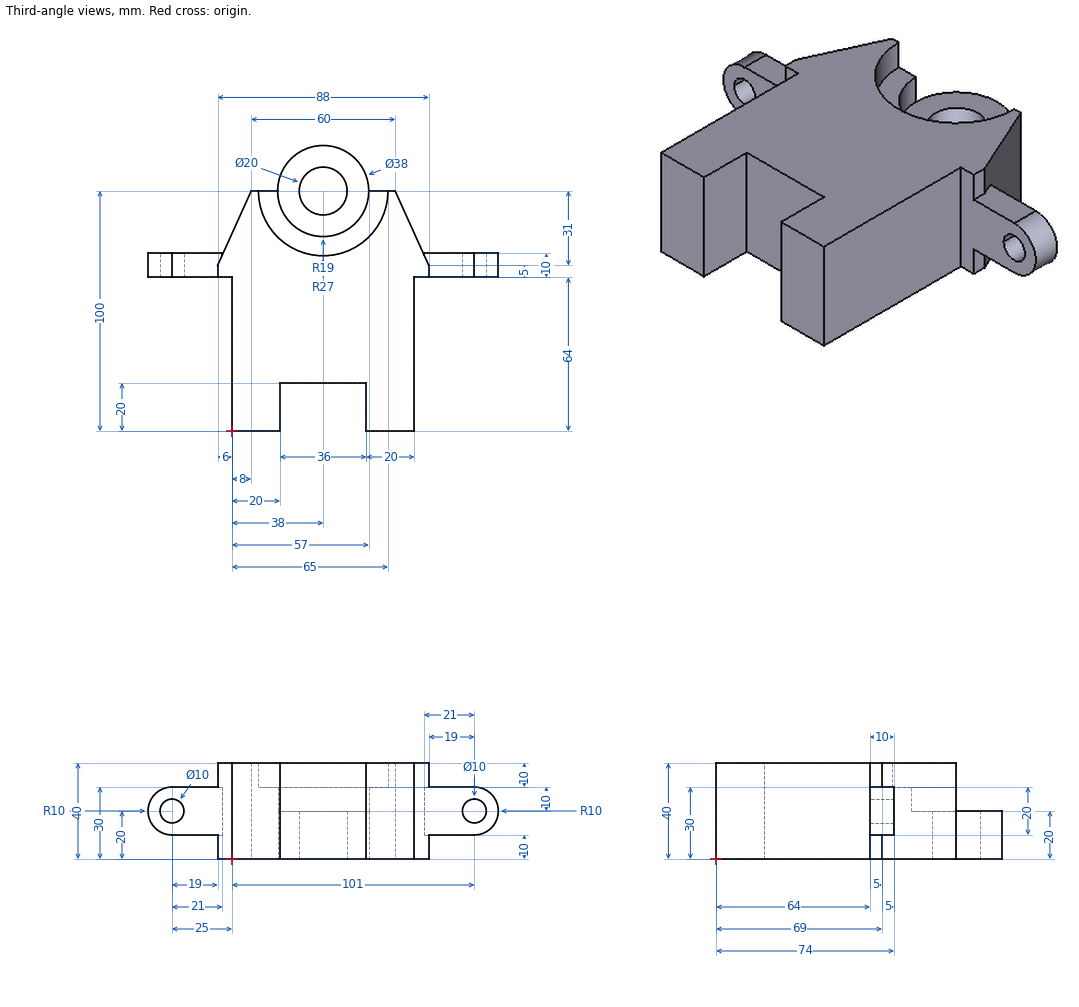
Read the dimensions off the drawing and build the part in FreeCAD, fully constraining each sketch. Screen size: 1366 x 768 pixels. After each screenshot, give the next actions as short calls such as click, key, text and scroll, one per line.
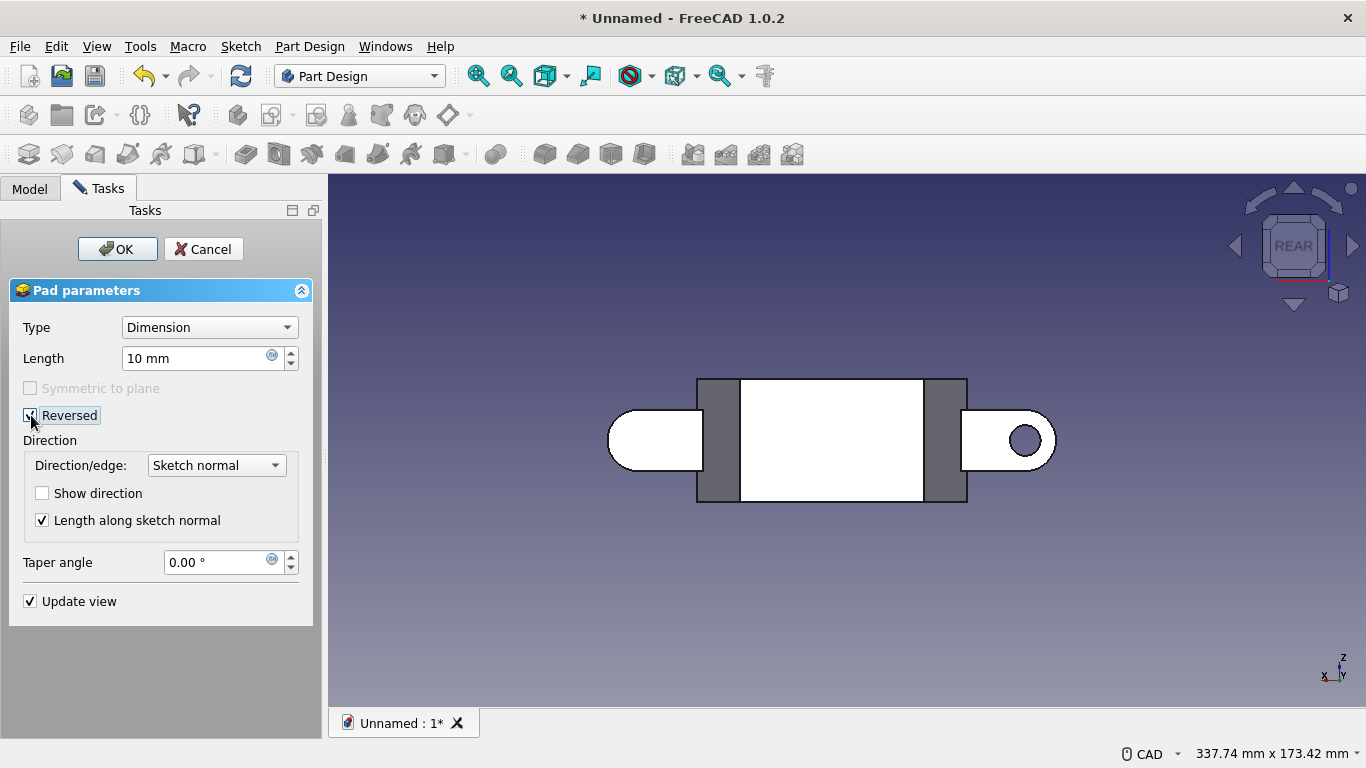
click(118, 249)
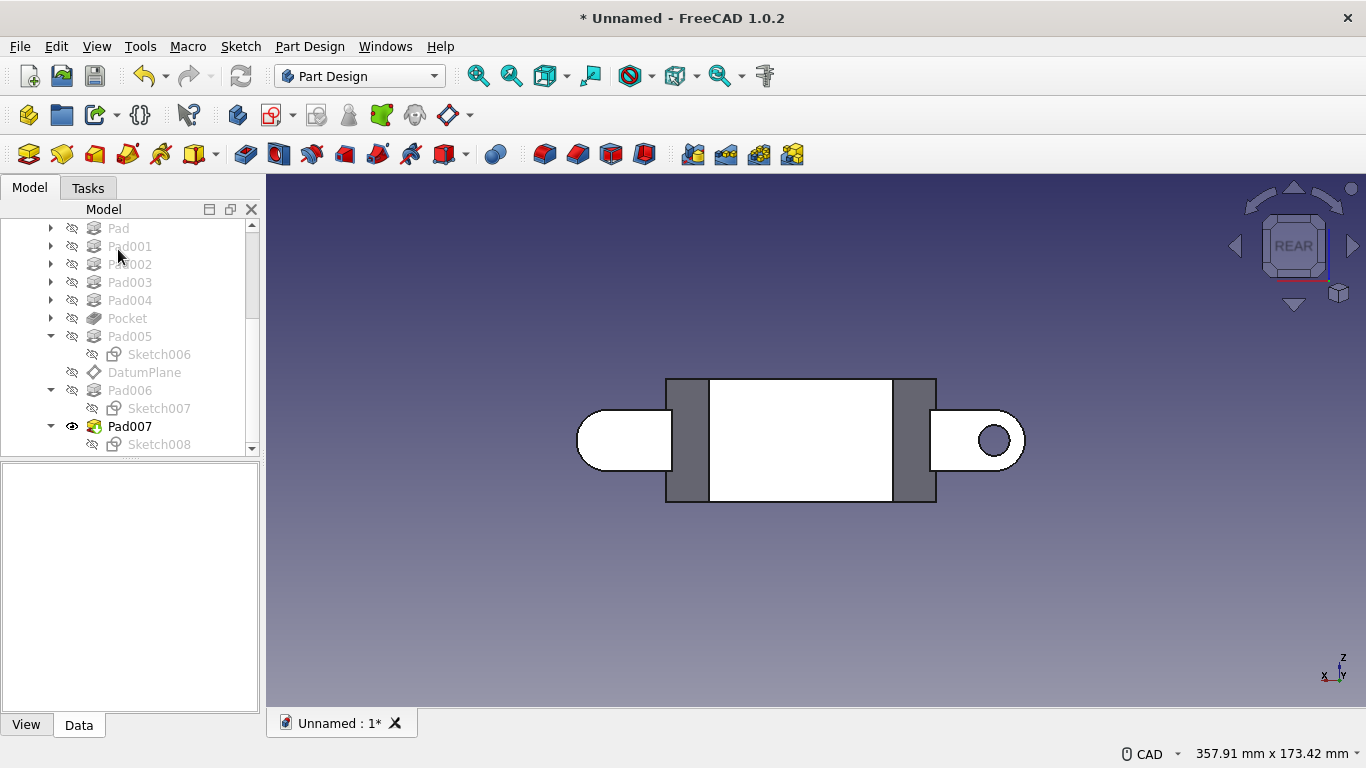
click(479, 76)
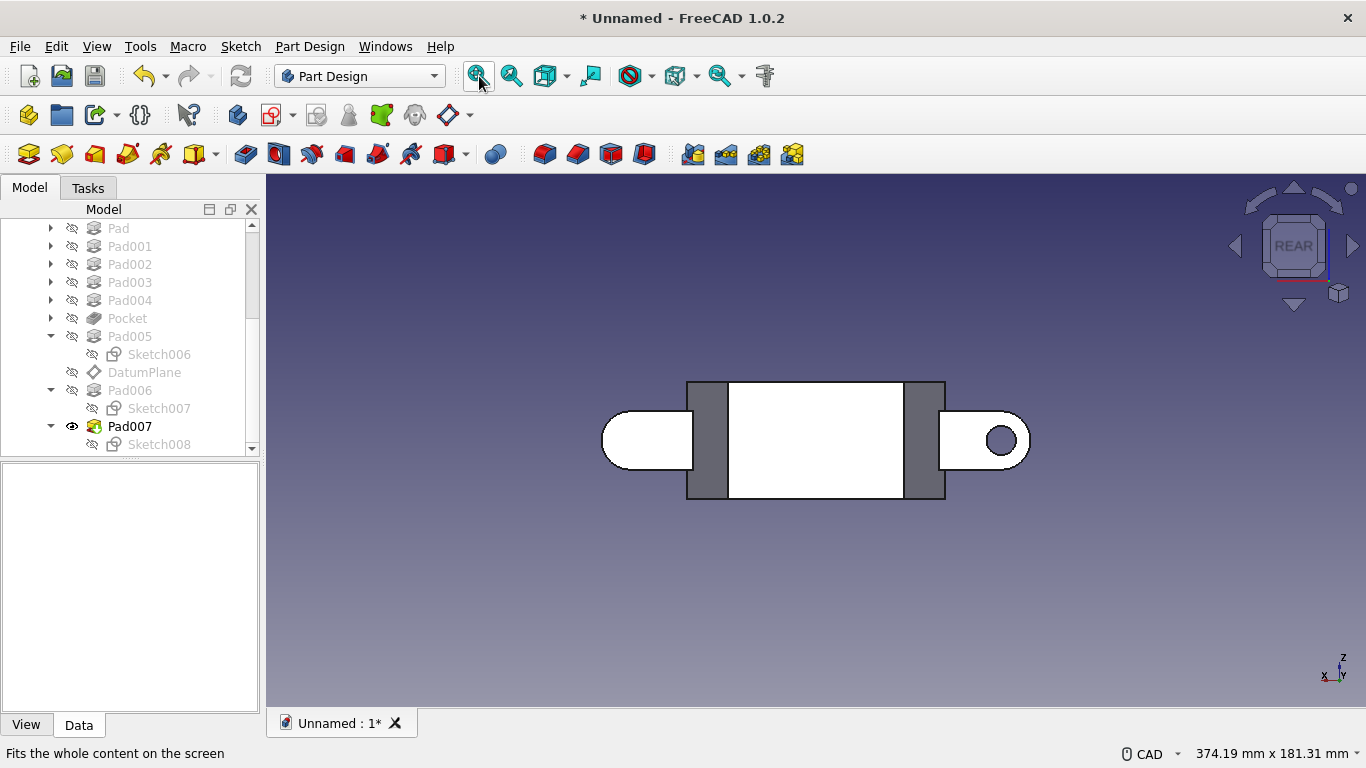
click(634, 439)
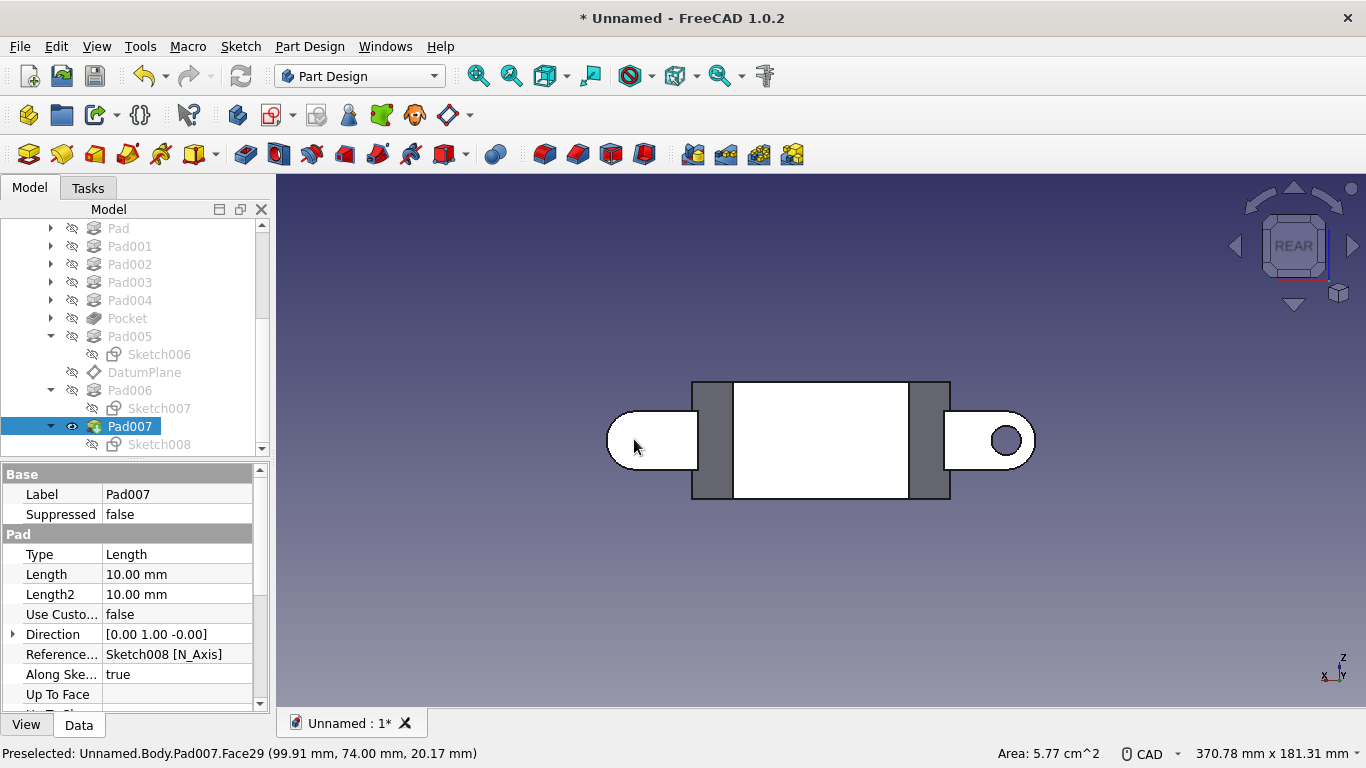
click(270, 116)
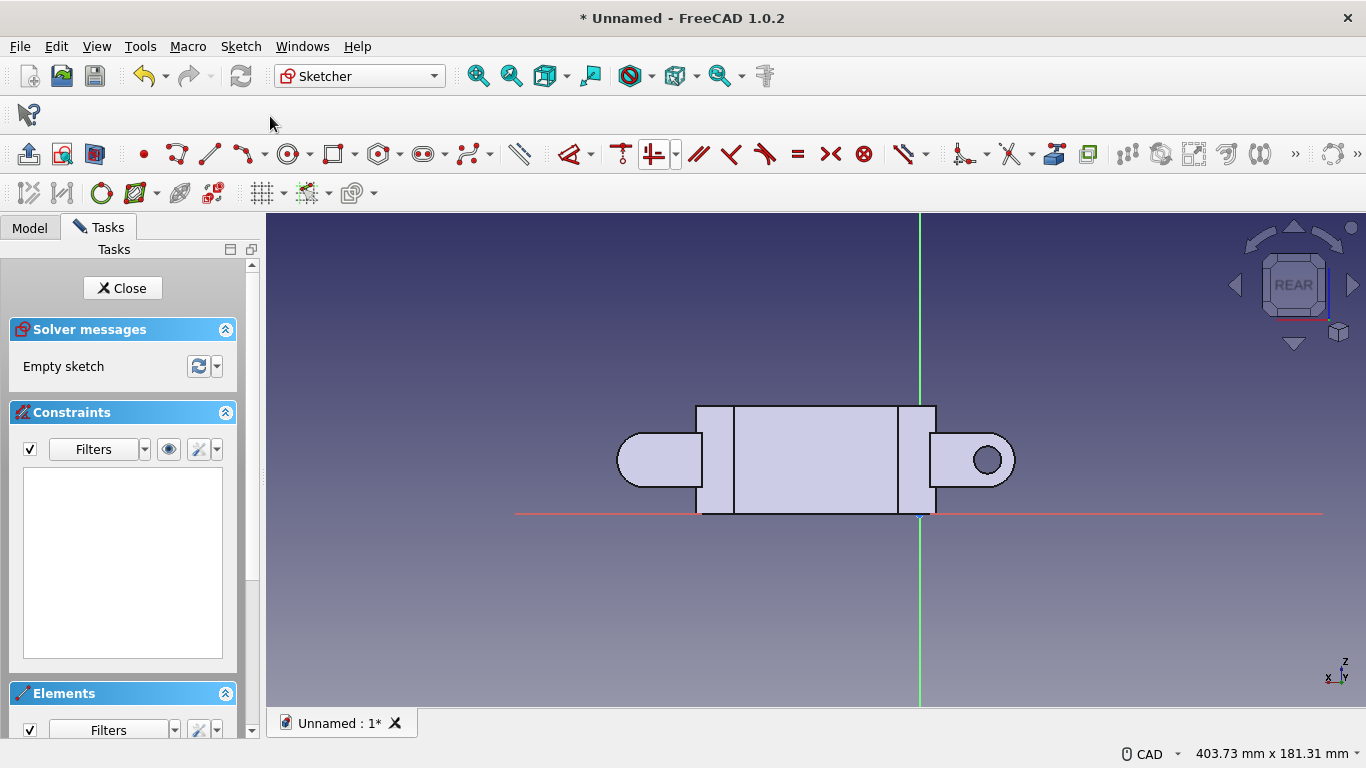
click(95, 154)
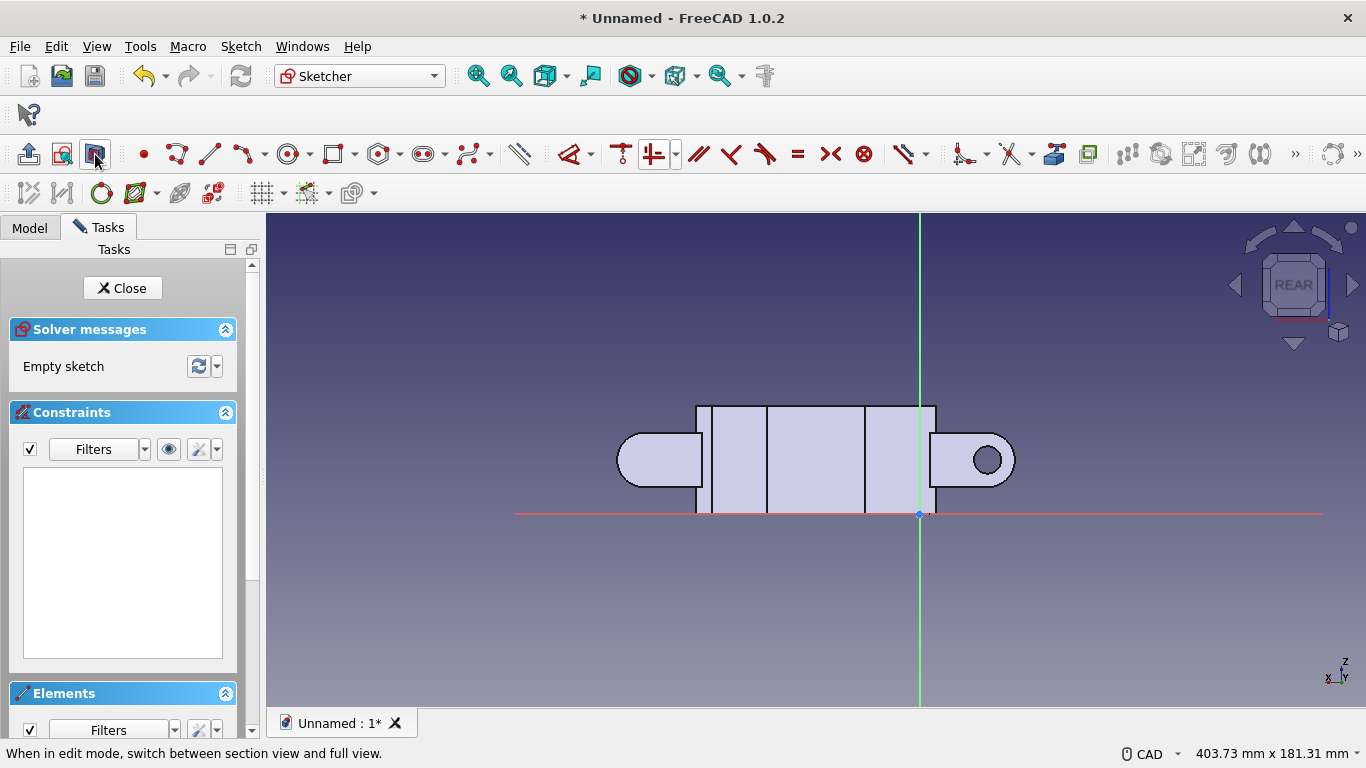
scroll(634, 460, up, 12)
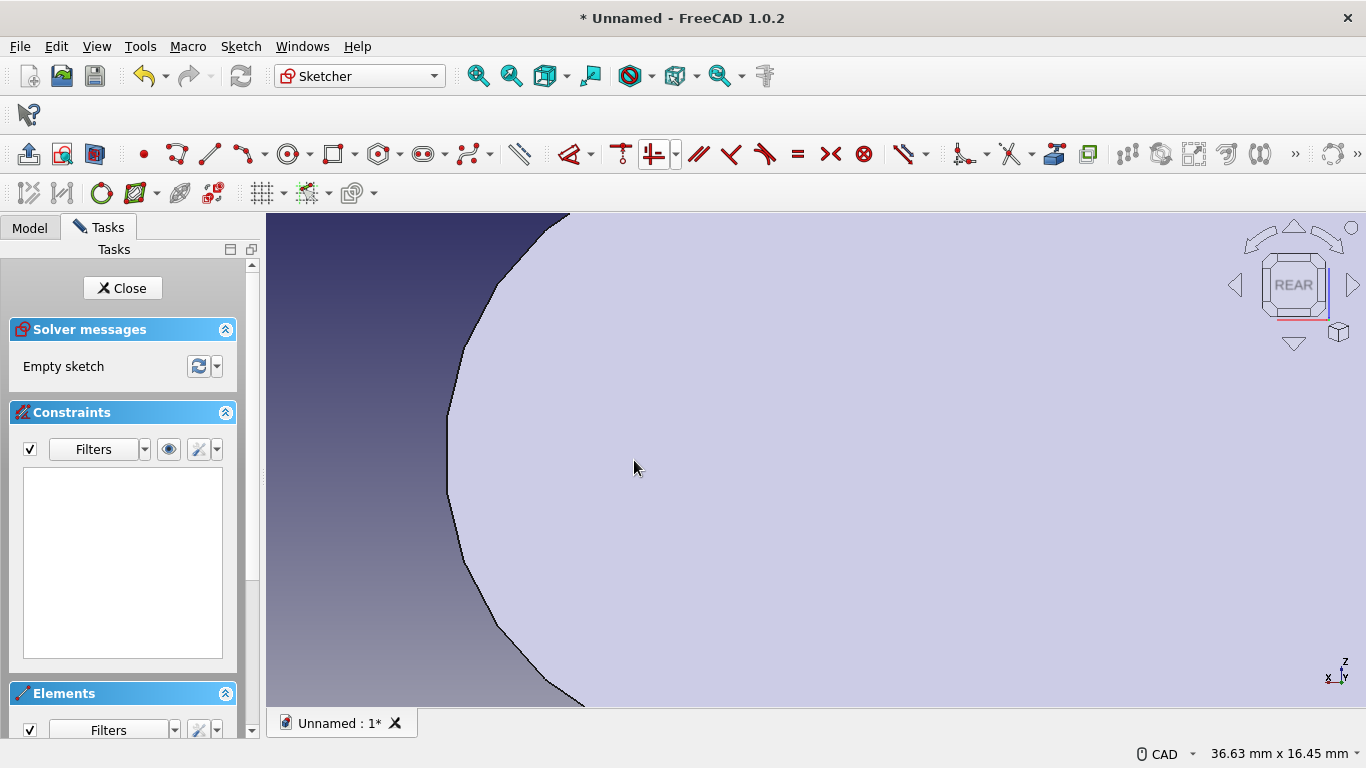
click(288, 154)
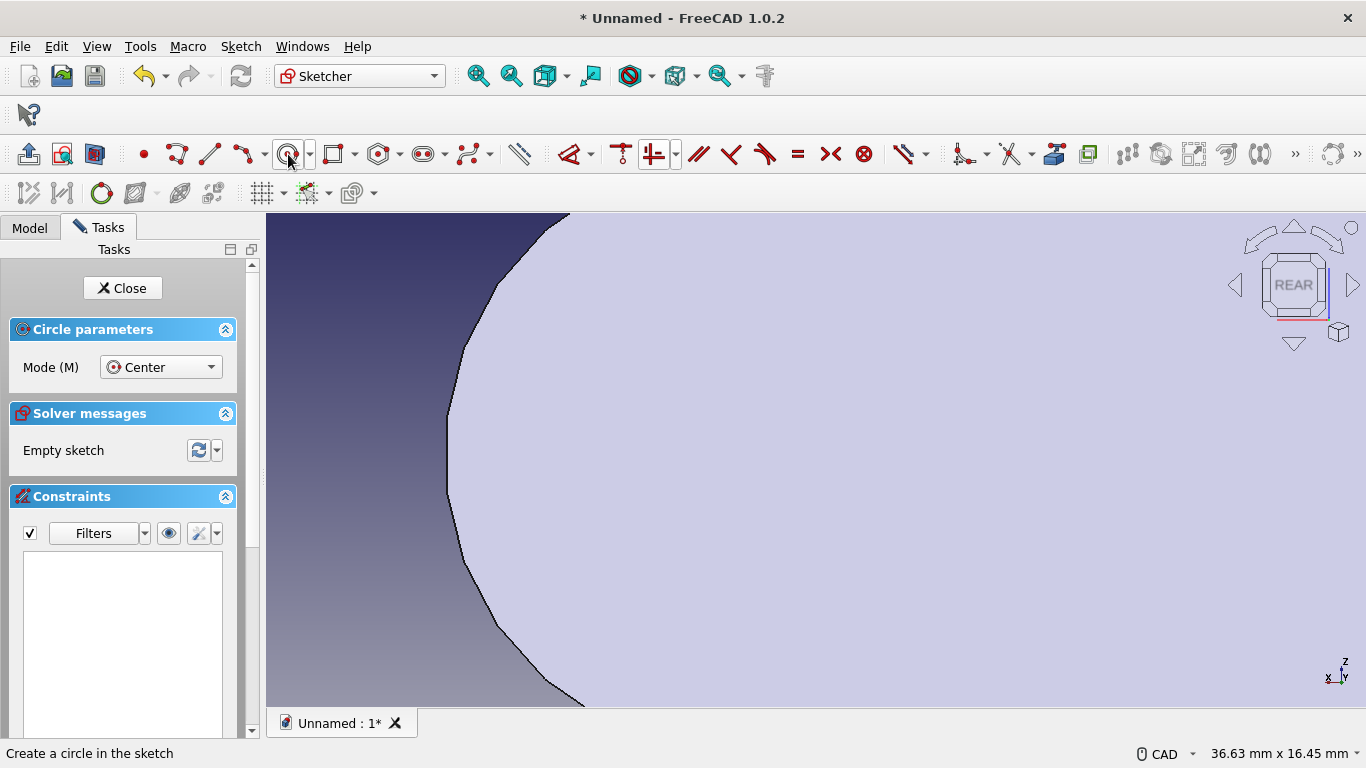
click(745, 455)
click(851, 349)
key(Escape)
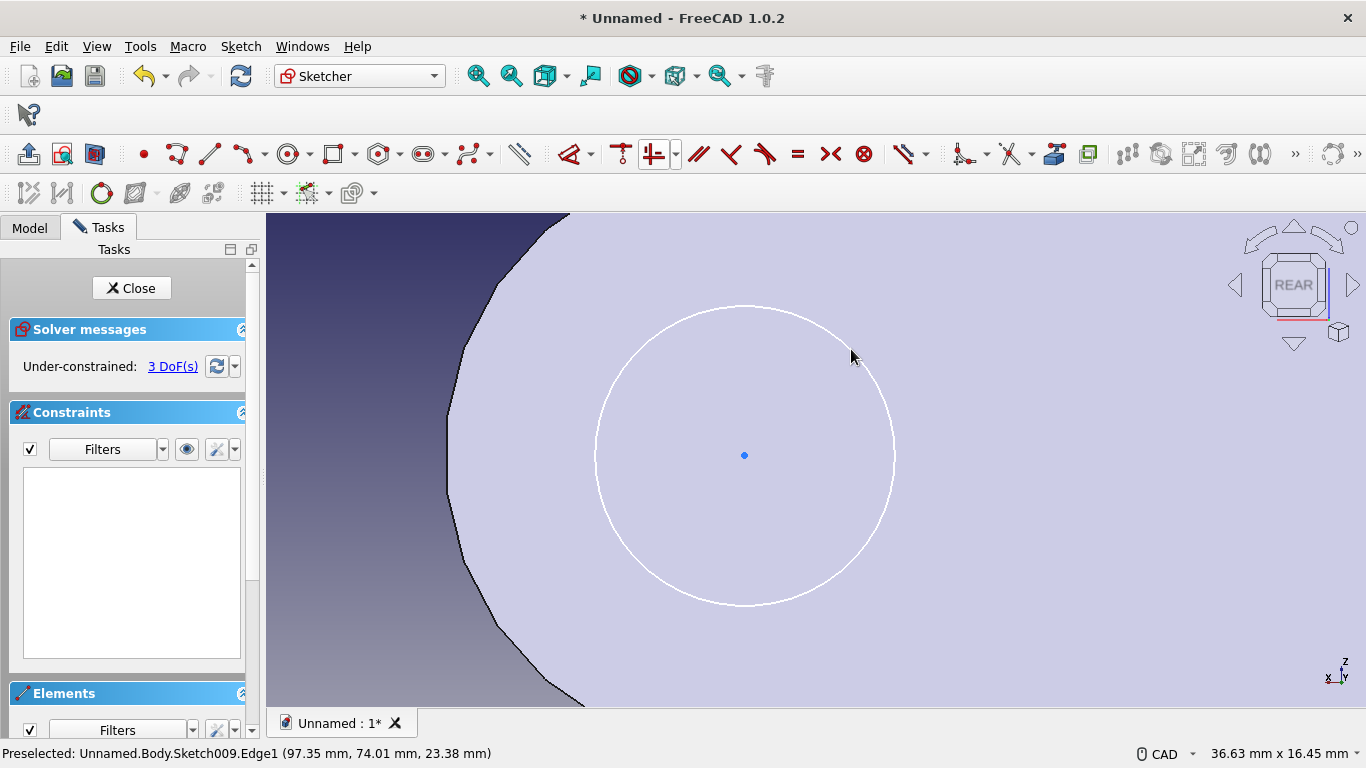
click(568, 154)